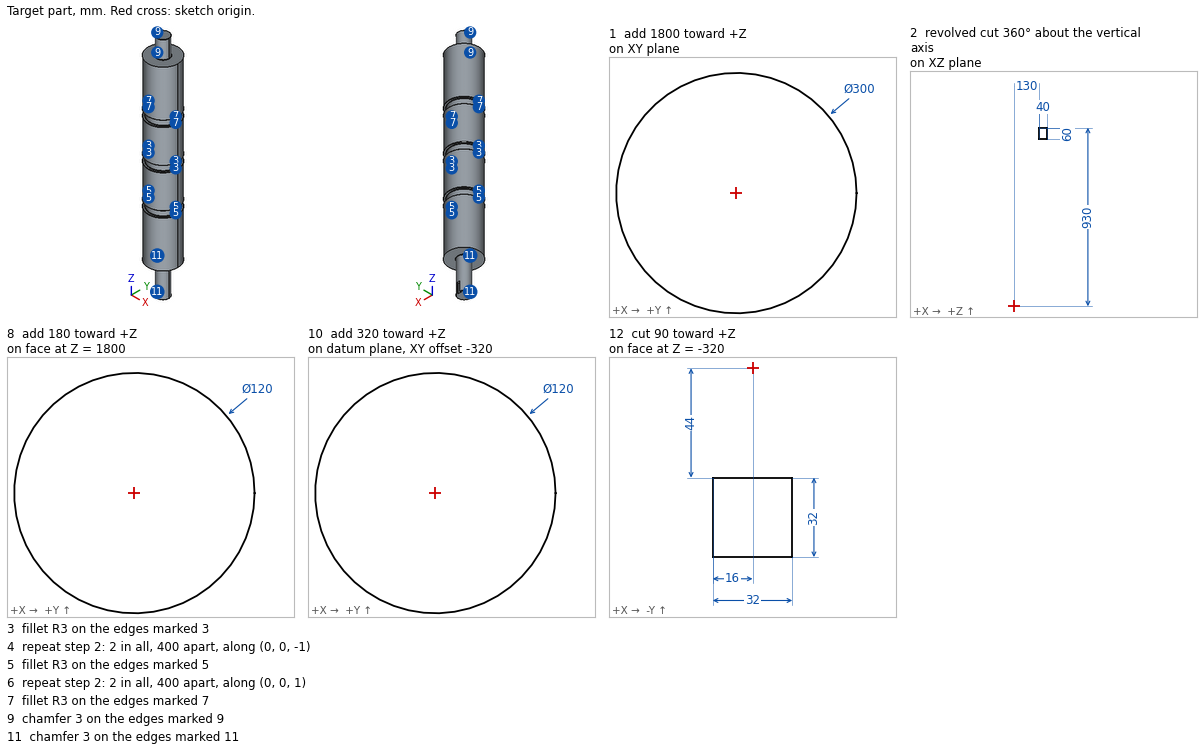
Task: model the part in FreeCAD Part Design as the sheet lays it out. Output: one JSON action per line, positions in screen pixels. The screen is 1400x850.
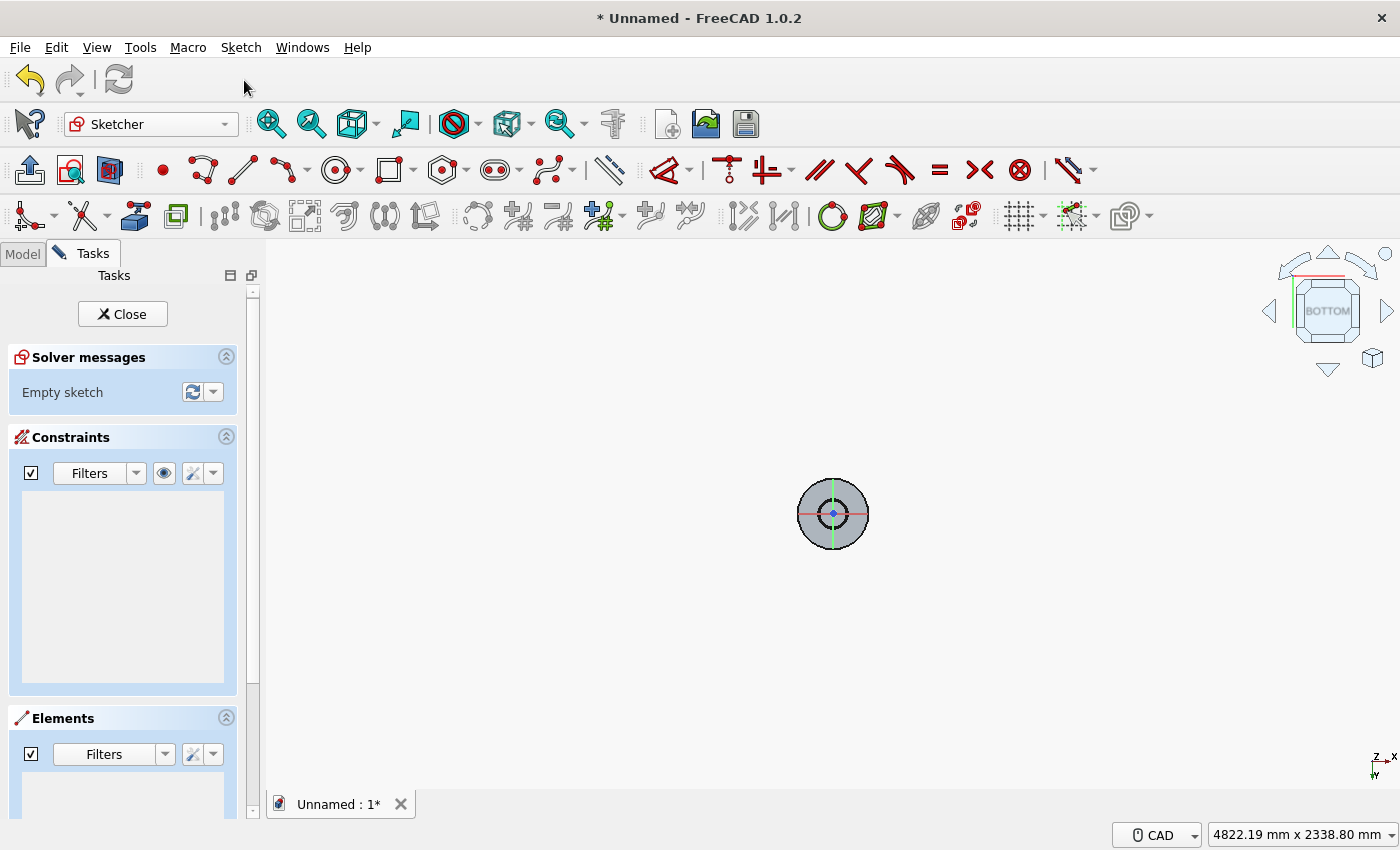
{"action": "scroll", "coordinate": [837, 523], "scroll_direction": "up", "scroll_amount": 15}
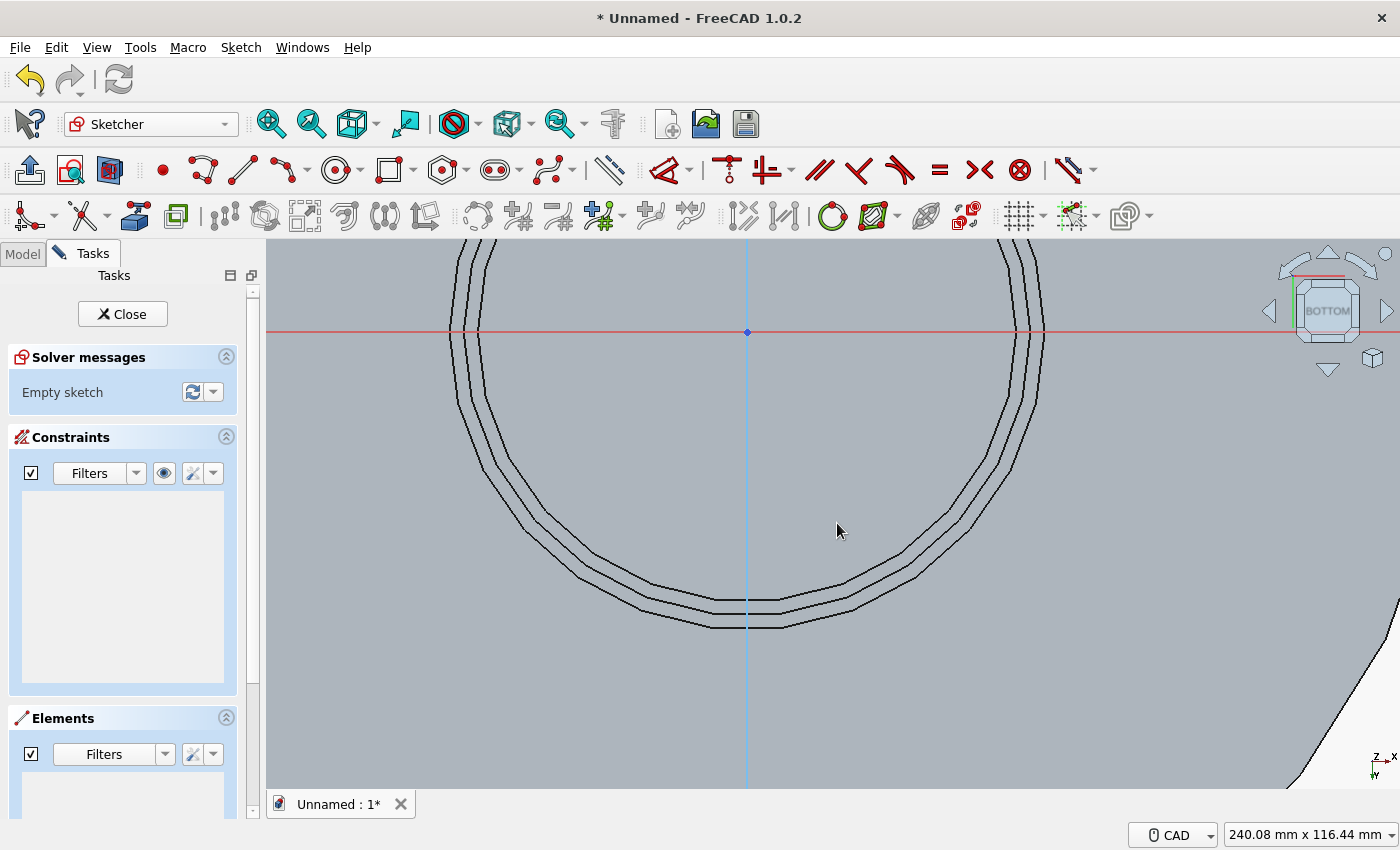
{"action": "left_click", "coordinate": [390, 170]}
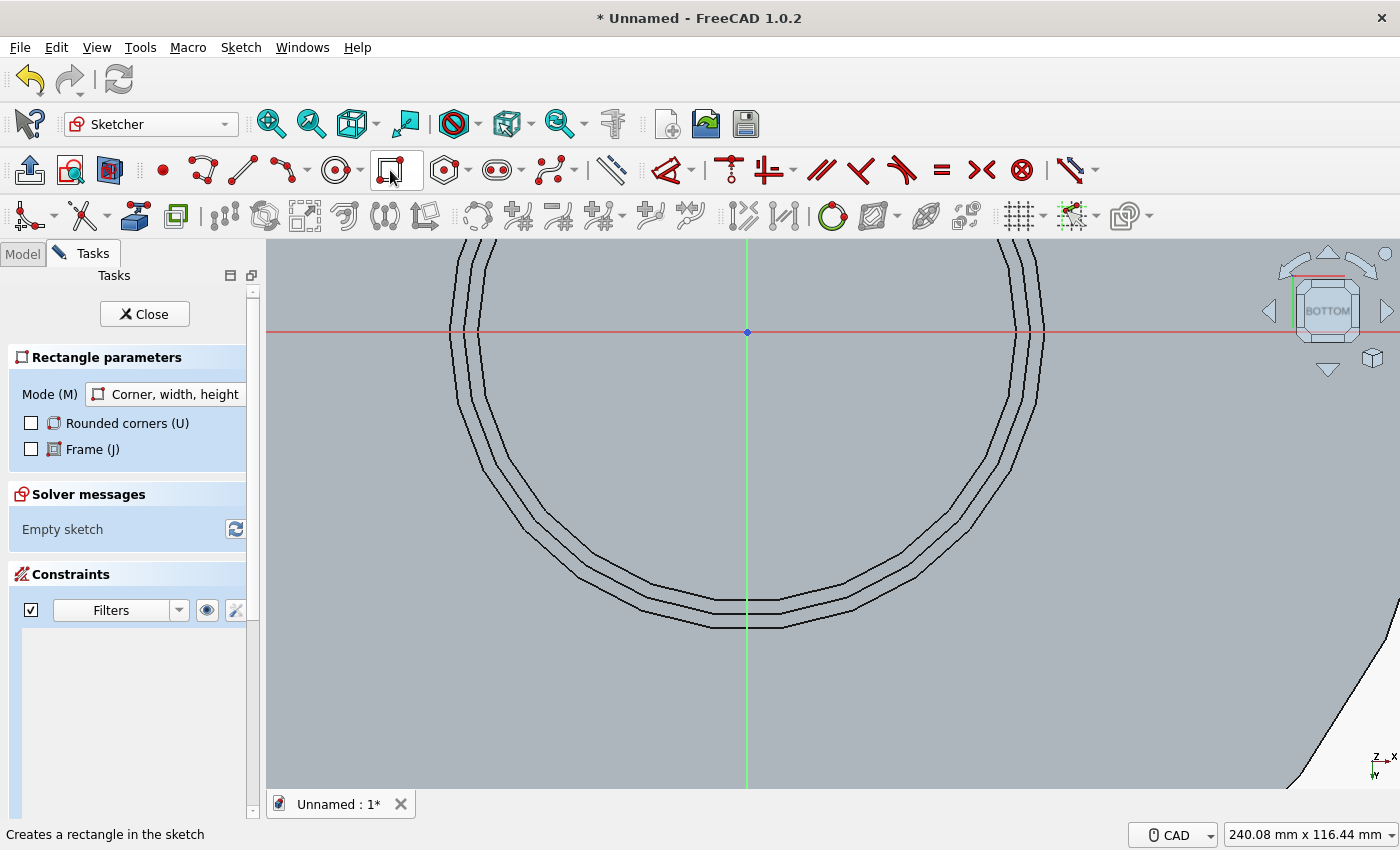
{"action": "left_click", "coordinate": [671, 540]}
{"action": "mouse_move", "coordinate": [823, 691]}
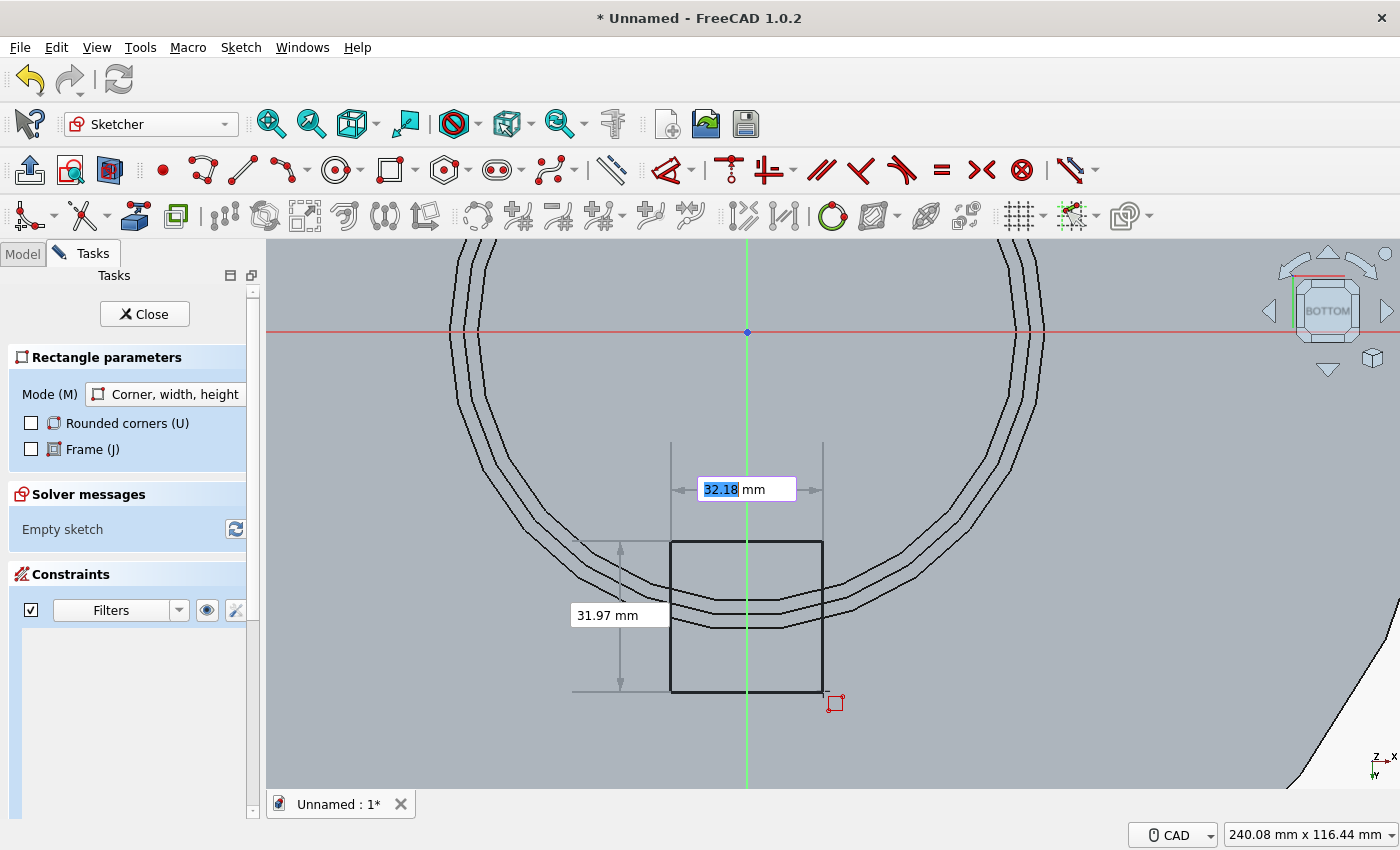
{"action": "type", "text": "32"}
{"action": "key", "text": "Tab"}
{"action": "type", "text": "32"}
{"action": "key", "text": "Return"}
{"action": "key", "text": "Escape"}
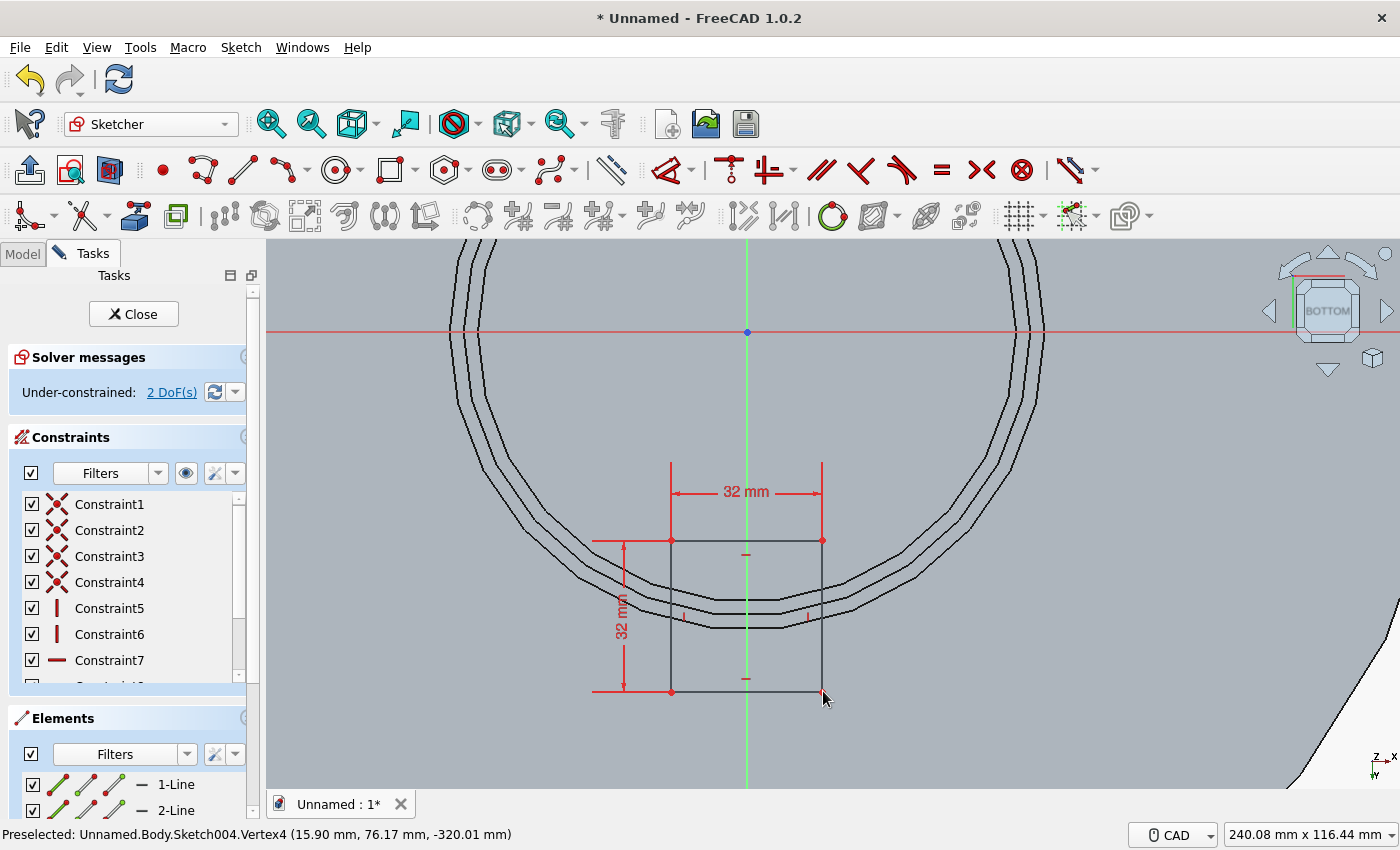
{"action": "left_click", "coordinate": [666, 170]}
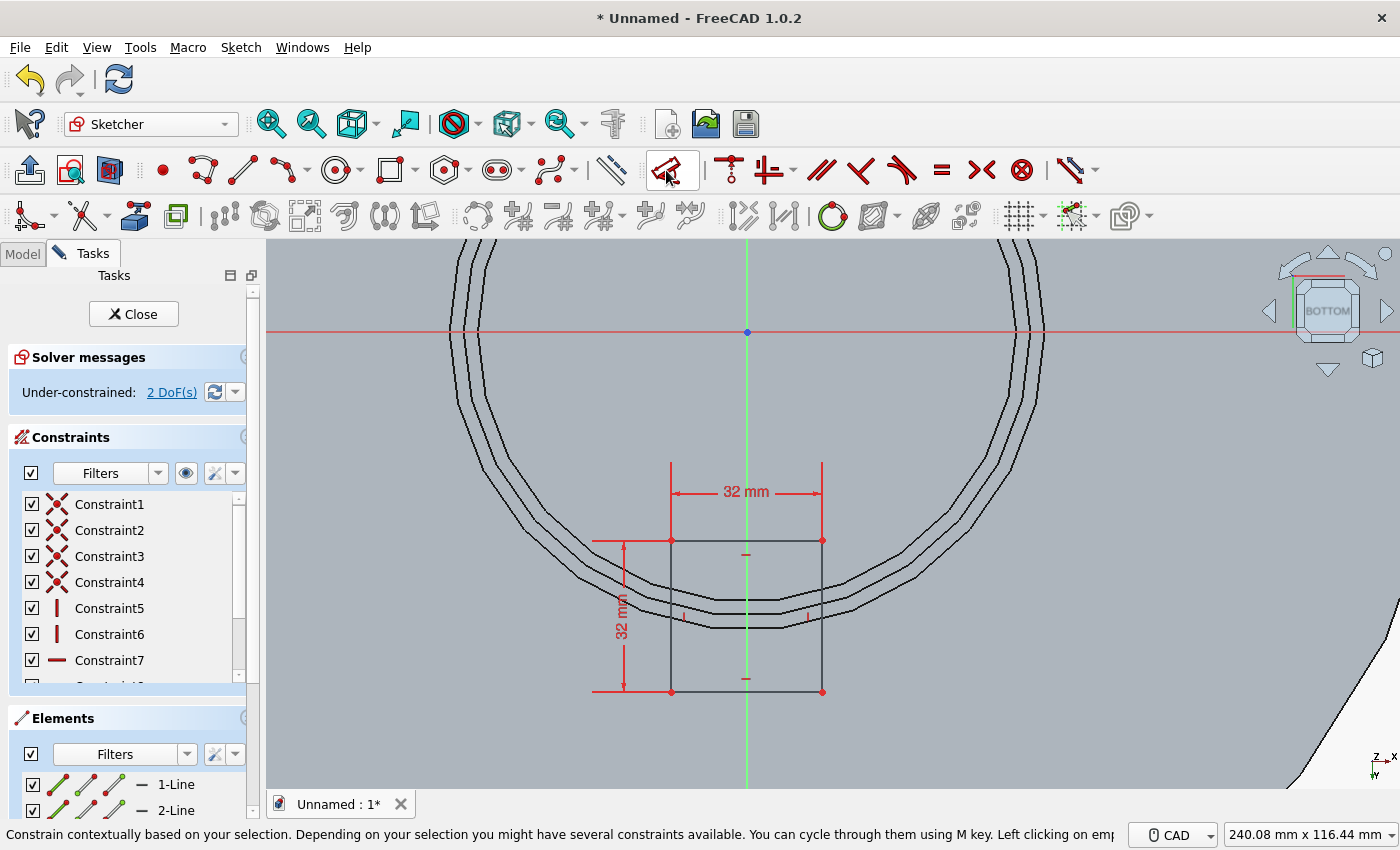
{"action": "left_click", "coordinate": [671, 541]}
{"action": "left_click", "coordinate": [709, 298]}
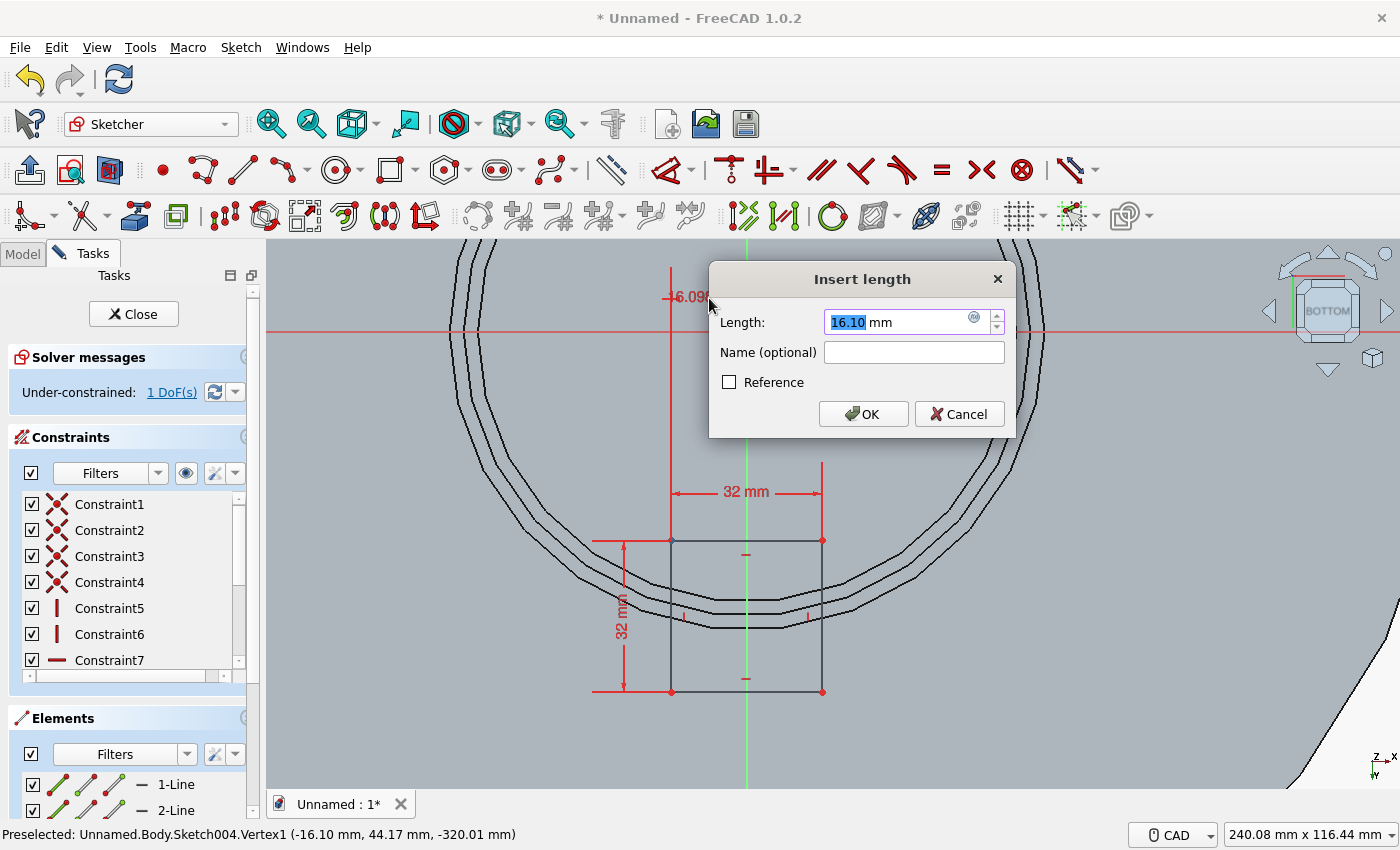
{"action": "type", "text": "16"}
{"action": "key", "text": "Return"}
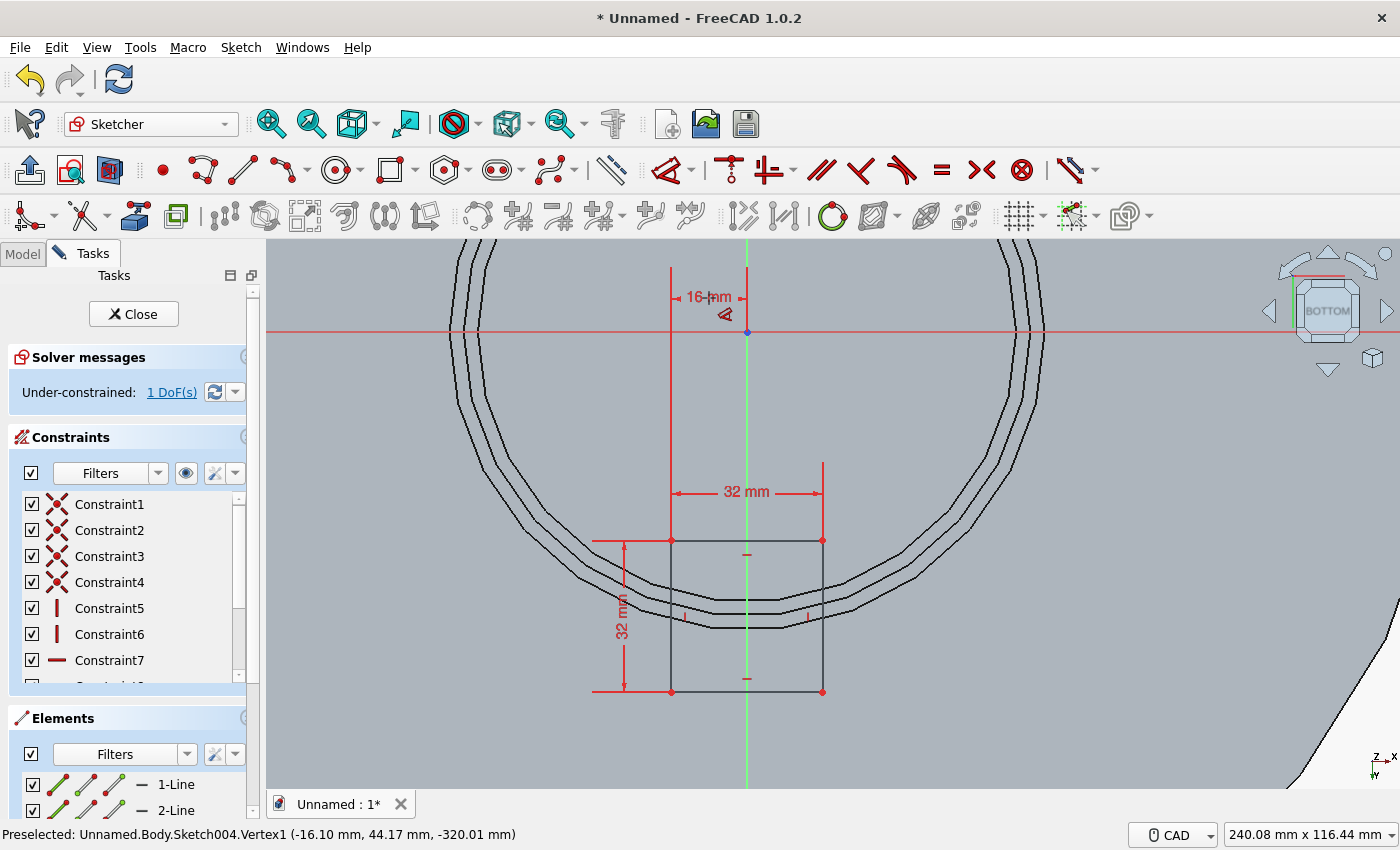
{"action": "left_click", "coordinate": [671, 541]}
{"action": "left_click", "coordinate": [637, 437]}